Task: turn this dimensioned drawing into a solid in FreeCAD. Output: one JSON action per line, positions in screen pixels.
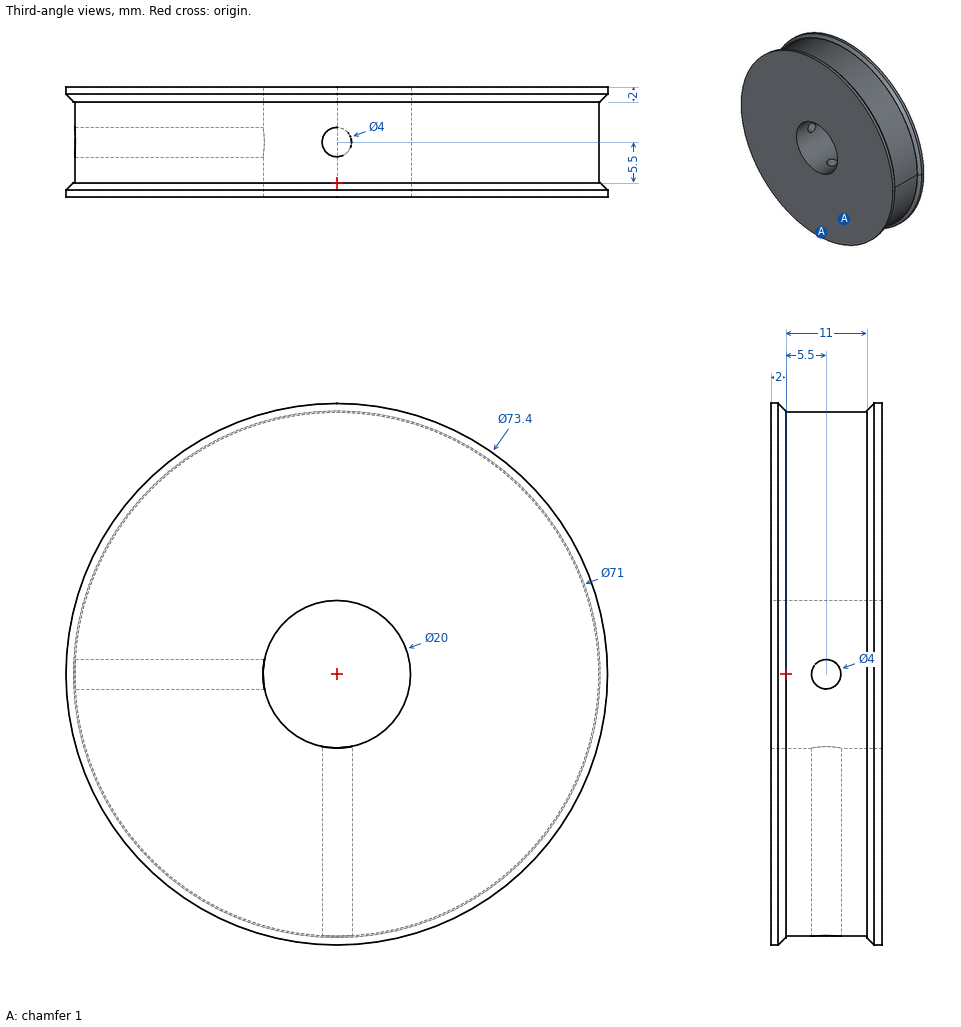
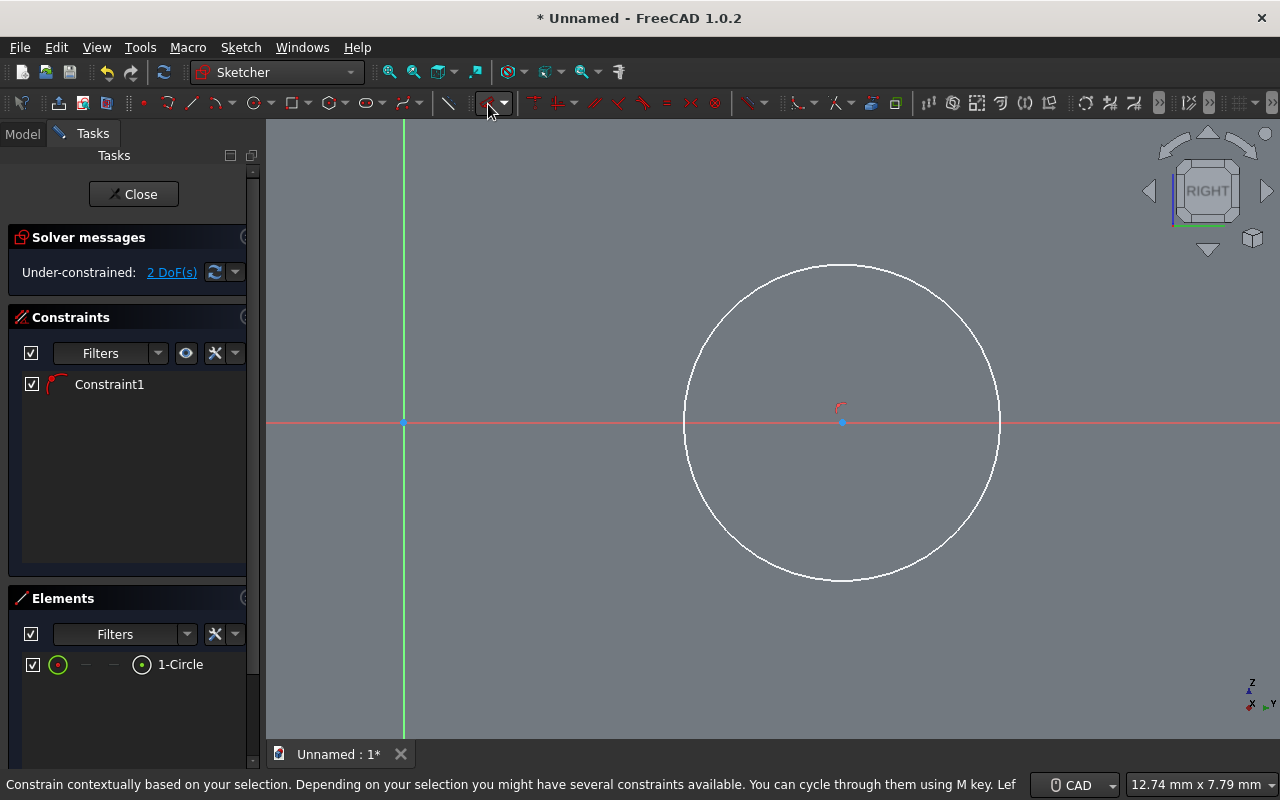
{"action": "left_click", "coordinate": [954, 311]}
{"action": "left_click", "coordinate": [977, 288]}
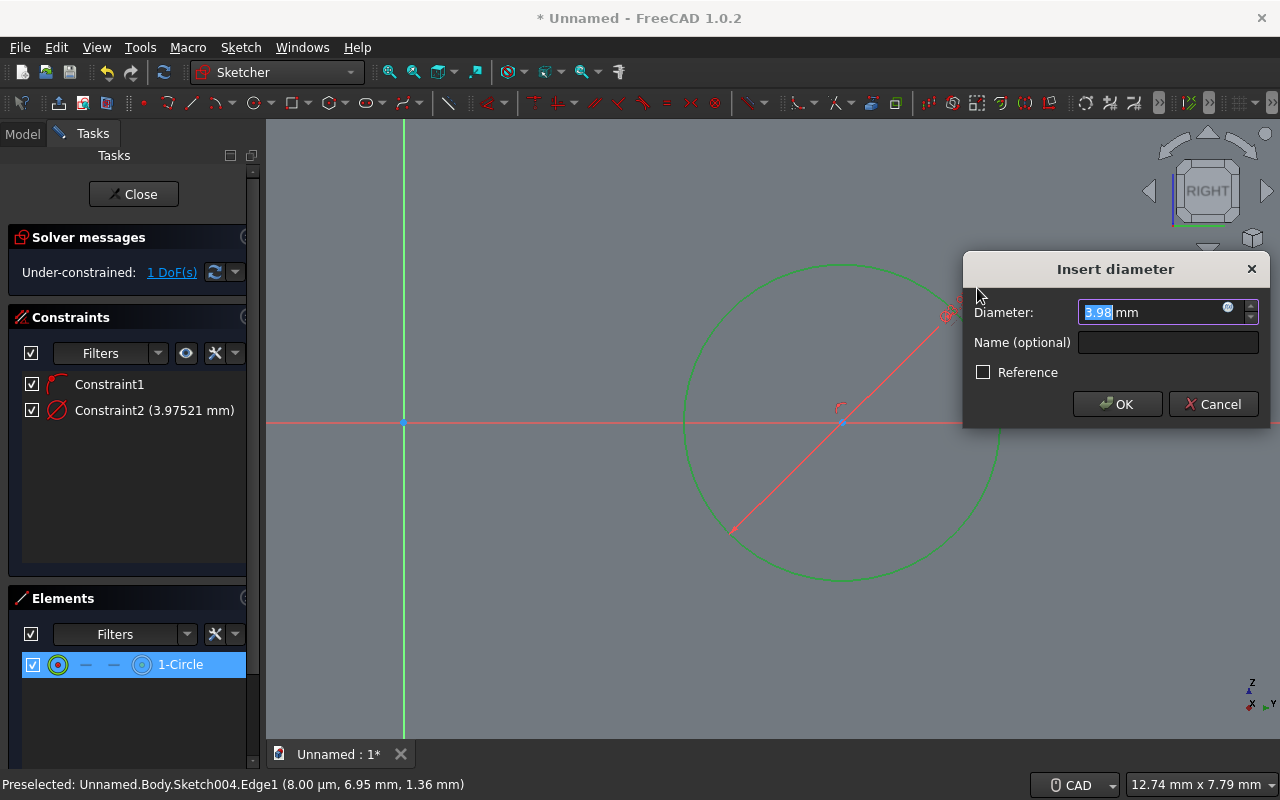
{"action": "type", "text": "4"}
{"action": "key", "text": "Return"}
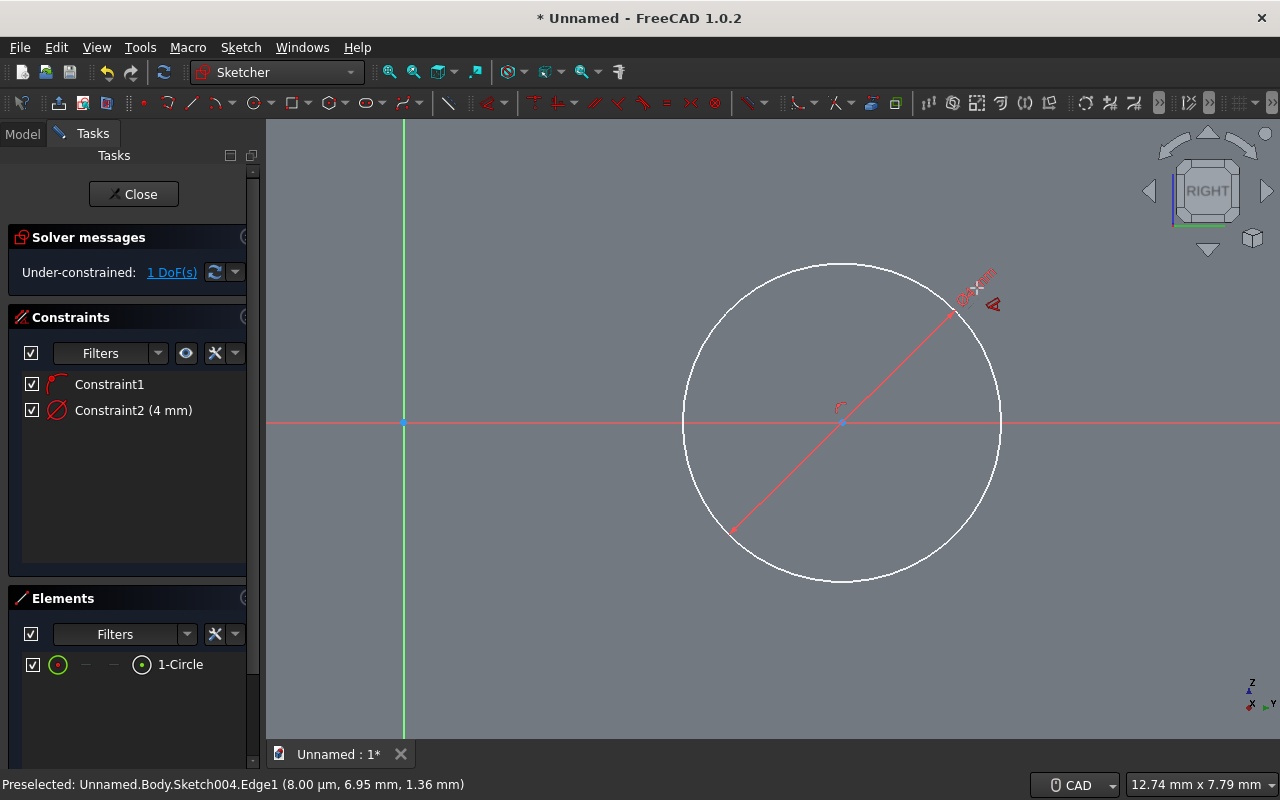
{"action": "left_click", "coordinate": [842, 423]}
{"action": "left_click", "coordinate": [623, 457]}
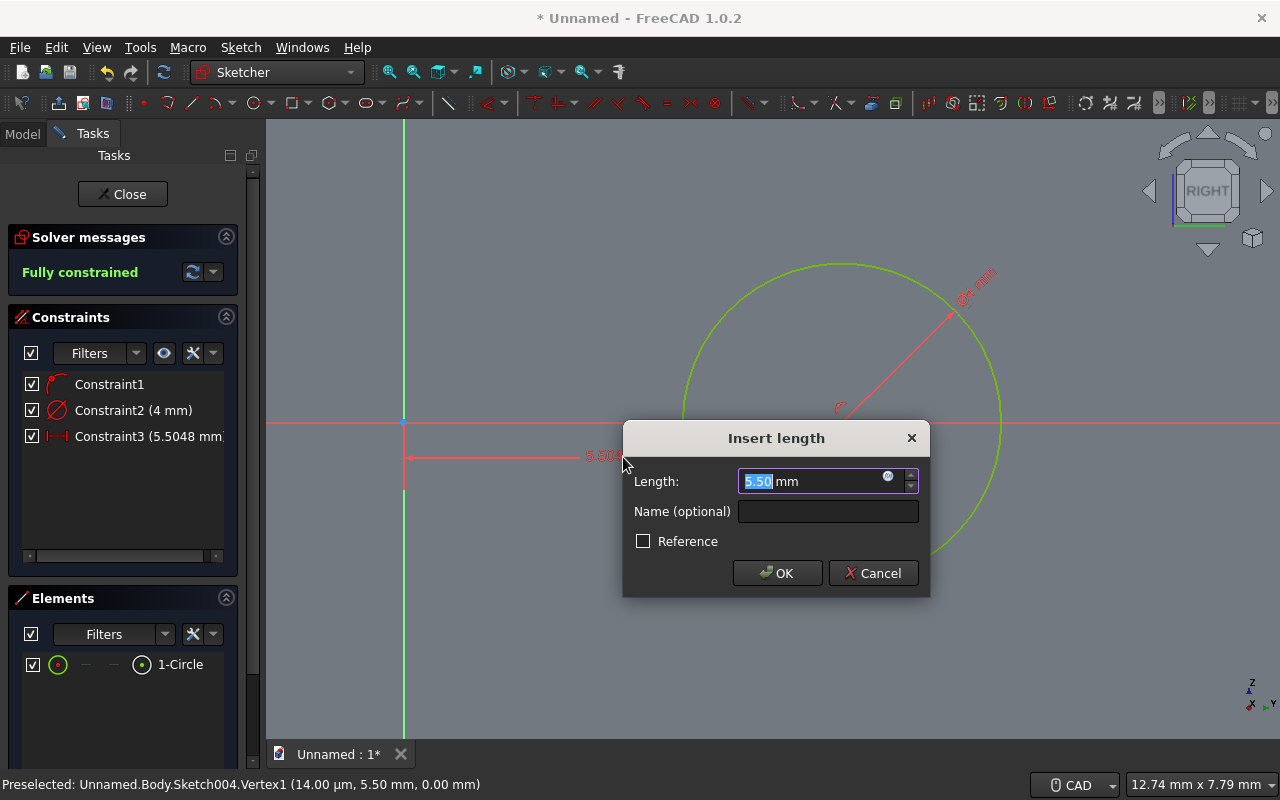
{"action": "type", "text": "5.5"}
{"action": "key", "text": "Return"}
{"action": "key", "text": "Escape"}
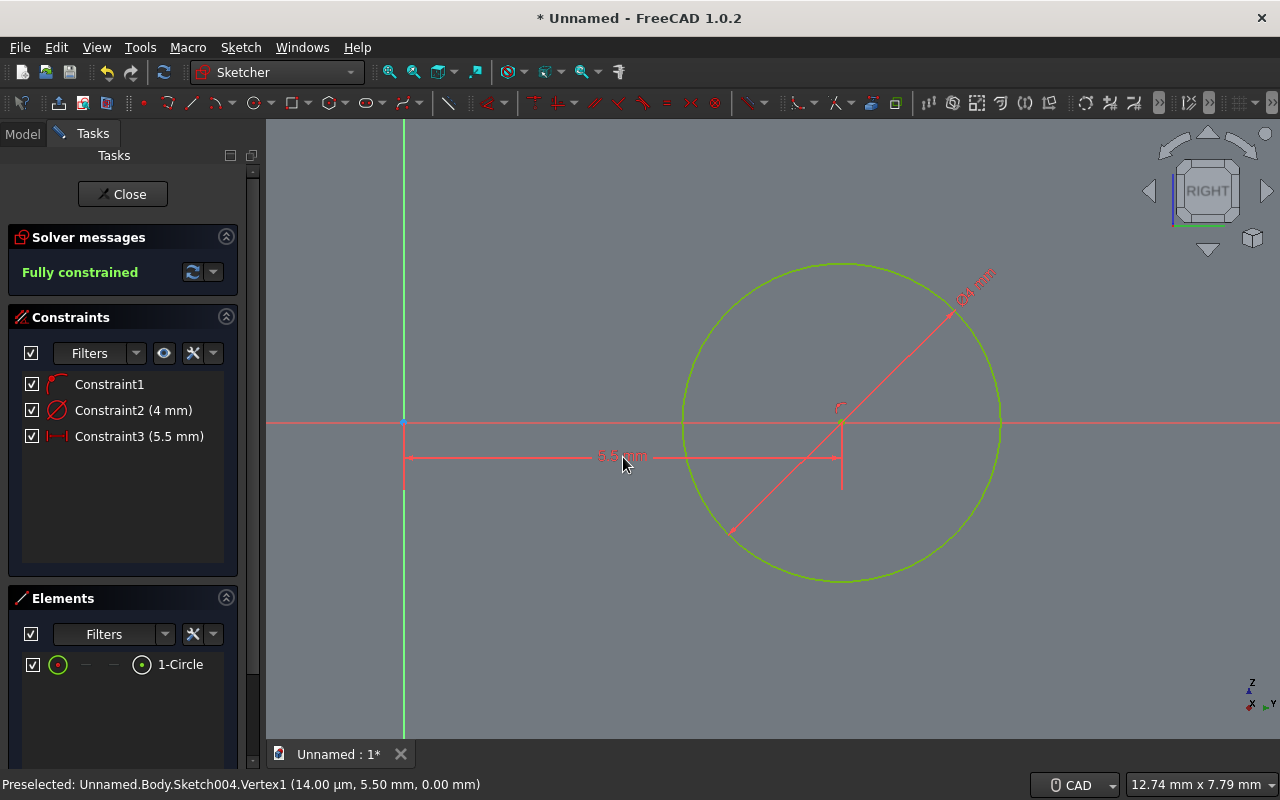
{"action": "left_click", "coordinate": [123, 194]}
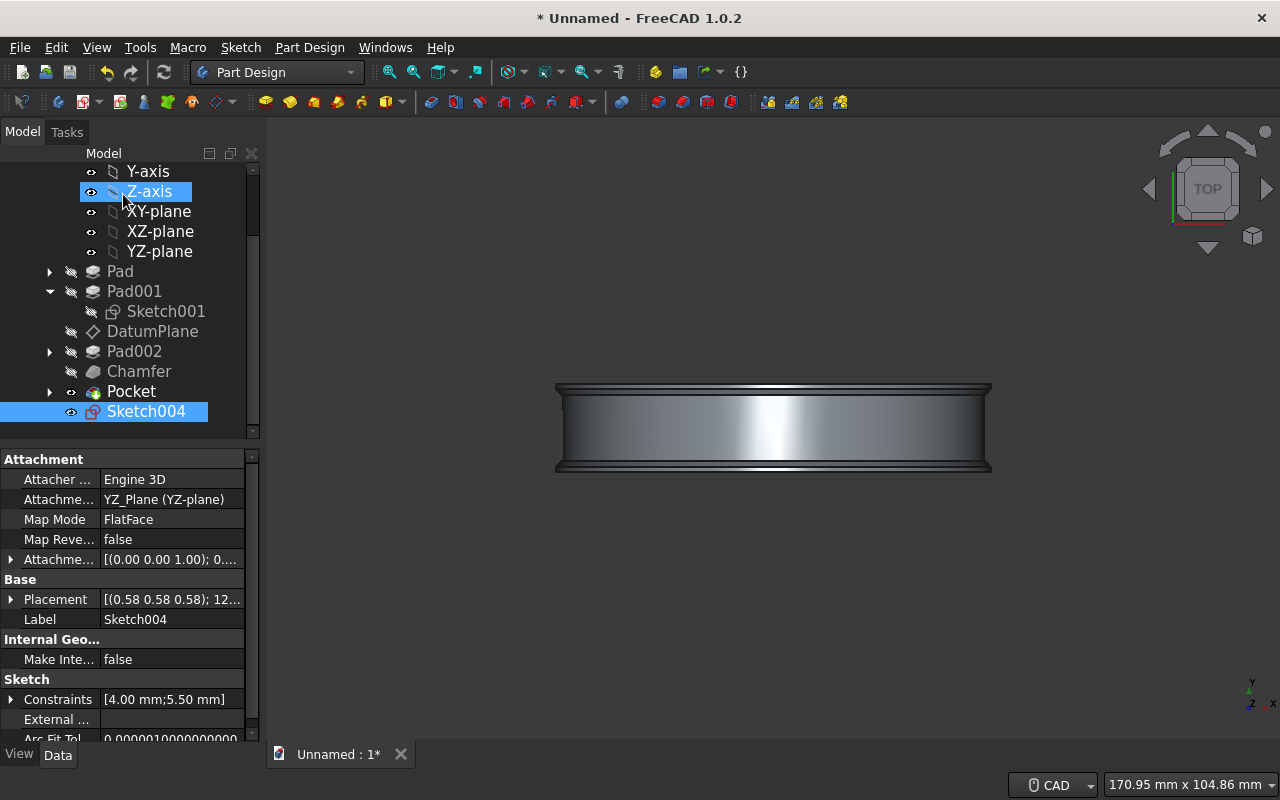
{"action": "left_click", "coordinate": [432, 102]}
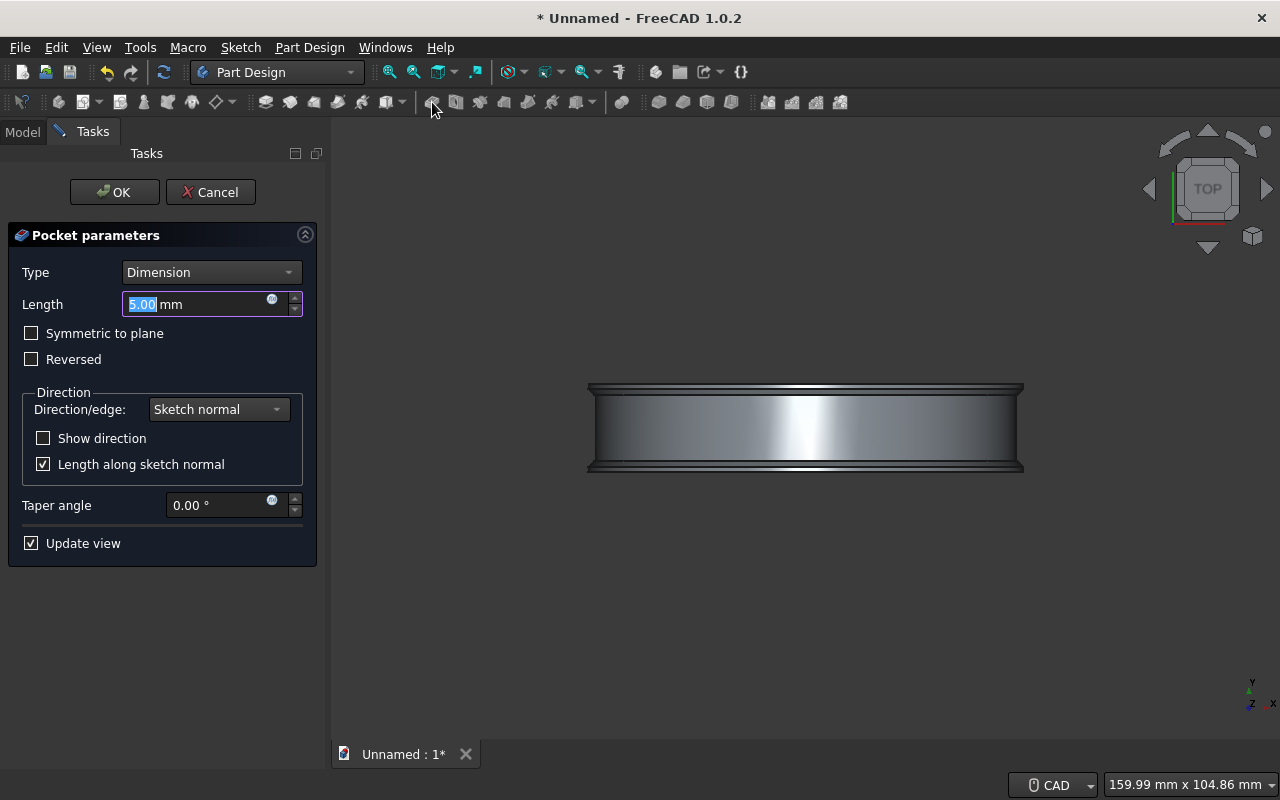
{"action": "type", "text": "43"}
{"action": "key", "text": "Tab"}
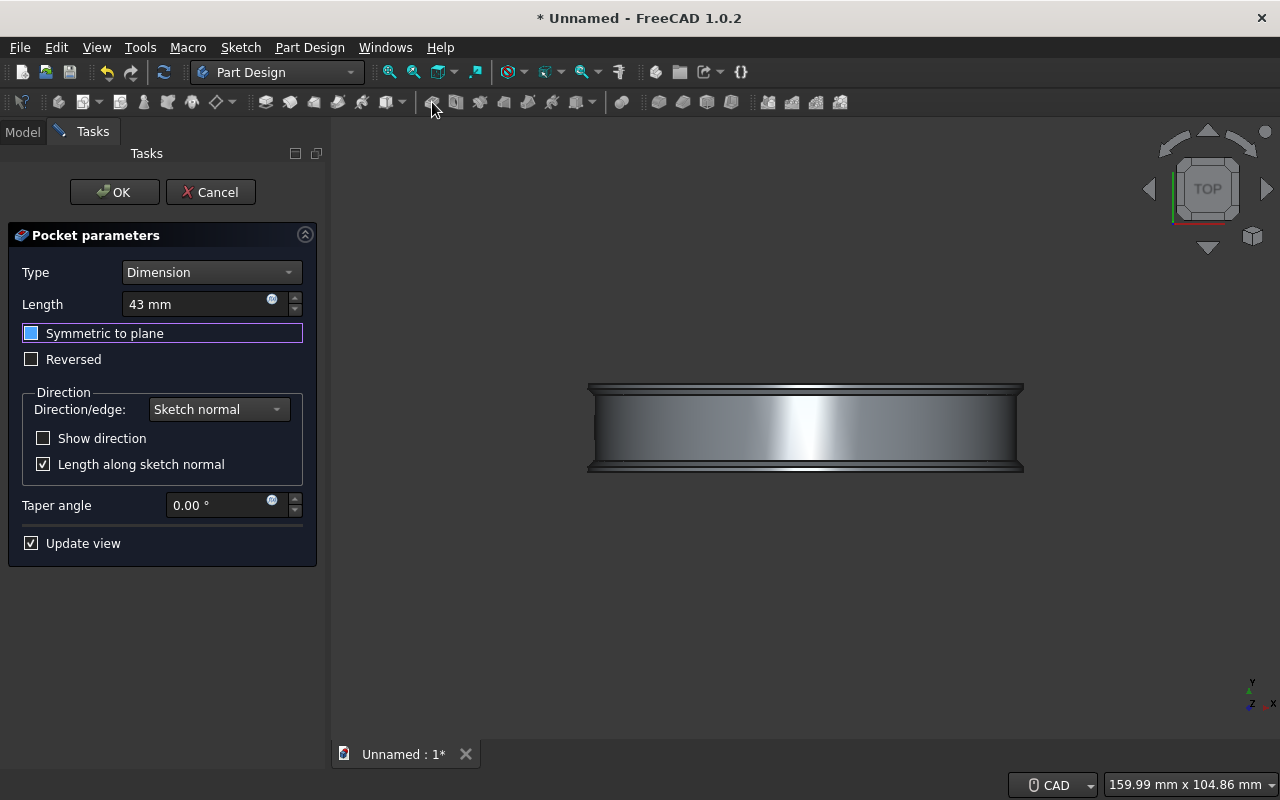
{"action": "left_click", "coordinate": [115, 192]}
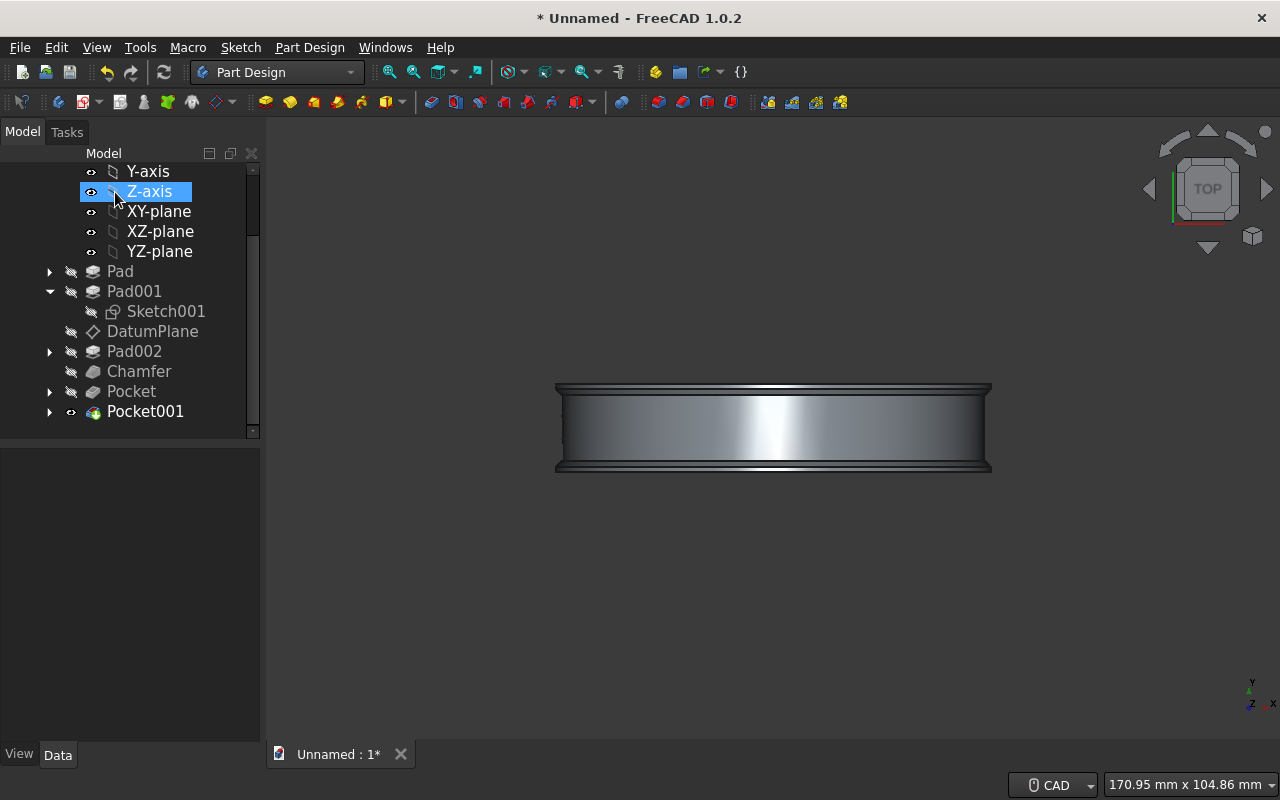
{"action": "key", "text": "0"}